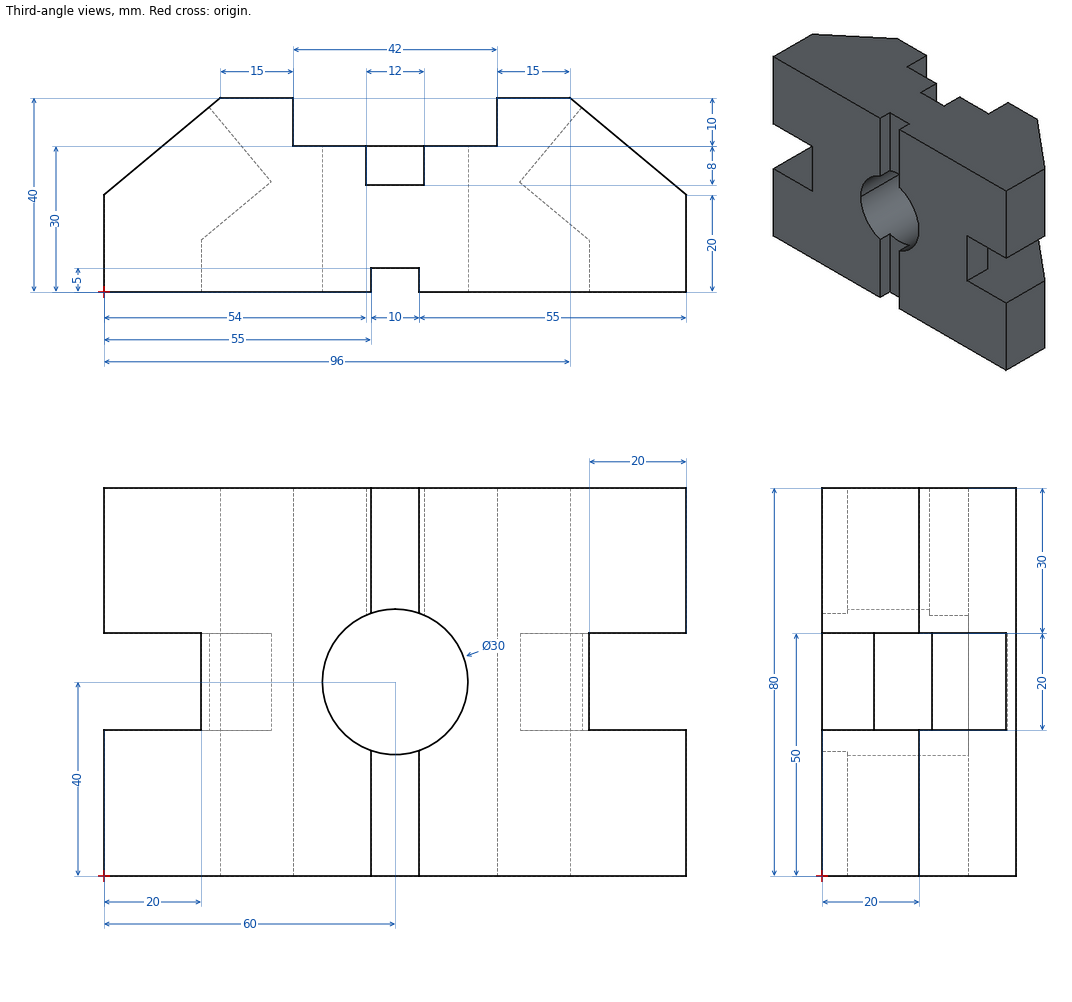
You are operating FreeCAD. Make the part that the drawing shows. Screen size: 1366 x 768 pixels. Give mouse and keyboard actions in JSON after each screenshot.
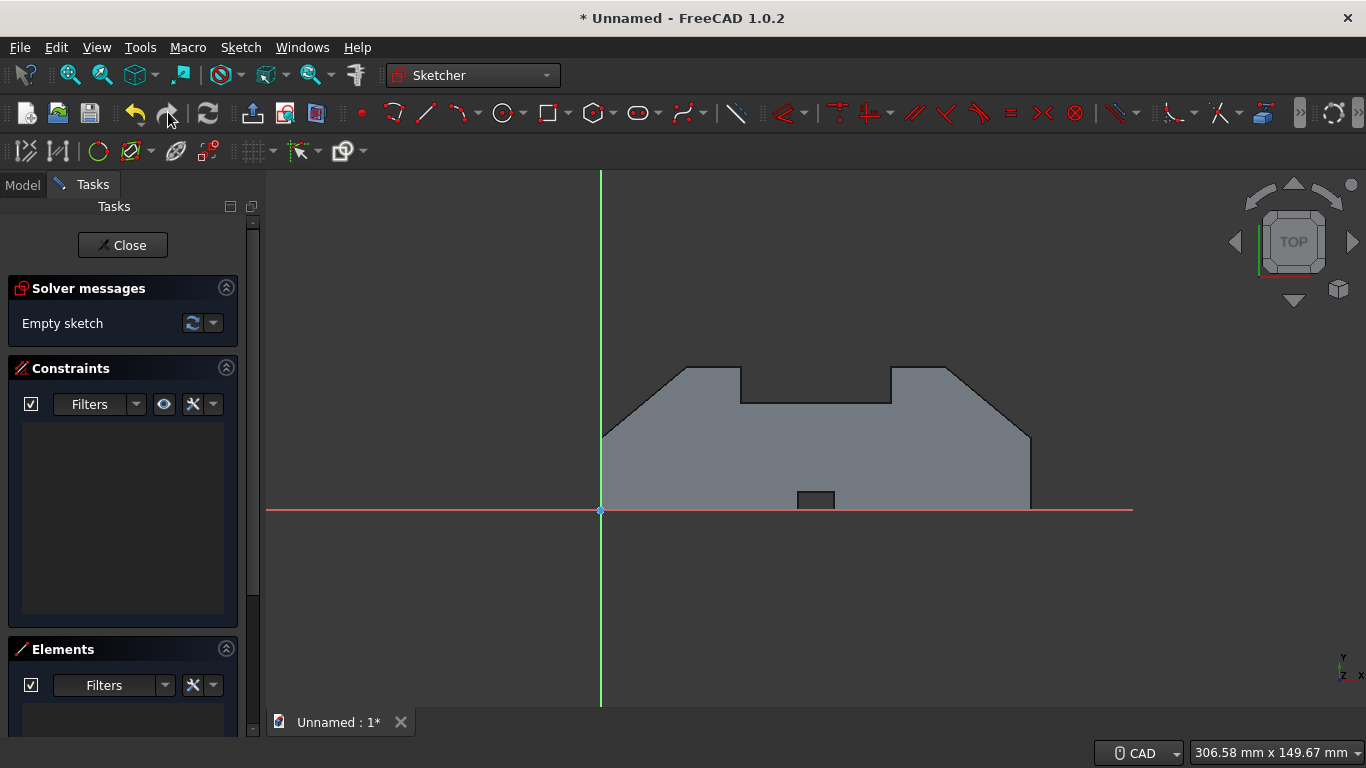
{"action": "scroll", "coordinate": [823, 415], "scroll_direction": "up", "scroll_amount": 12}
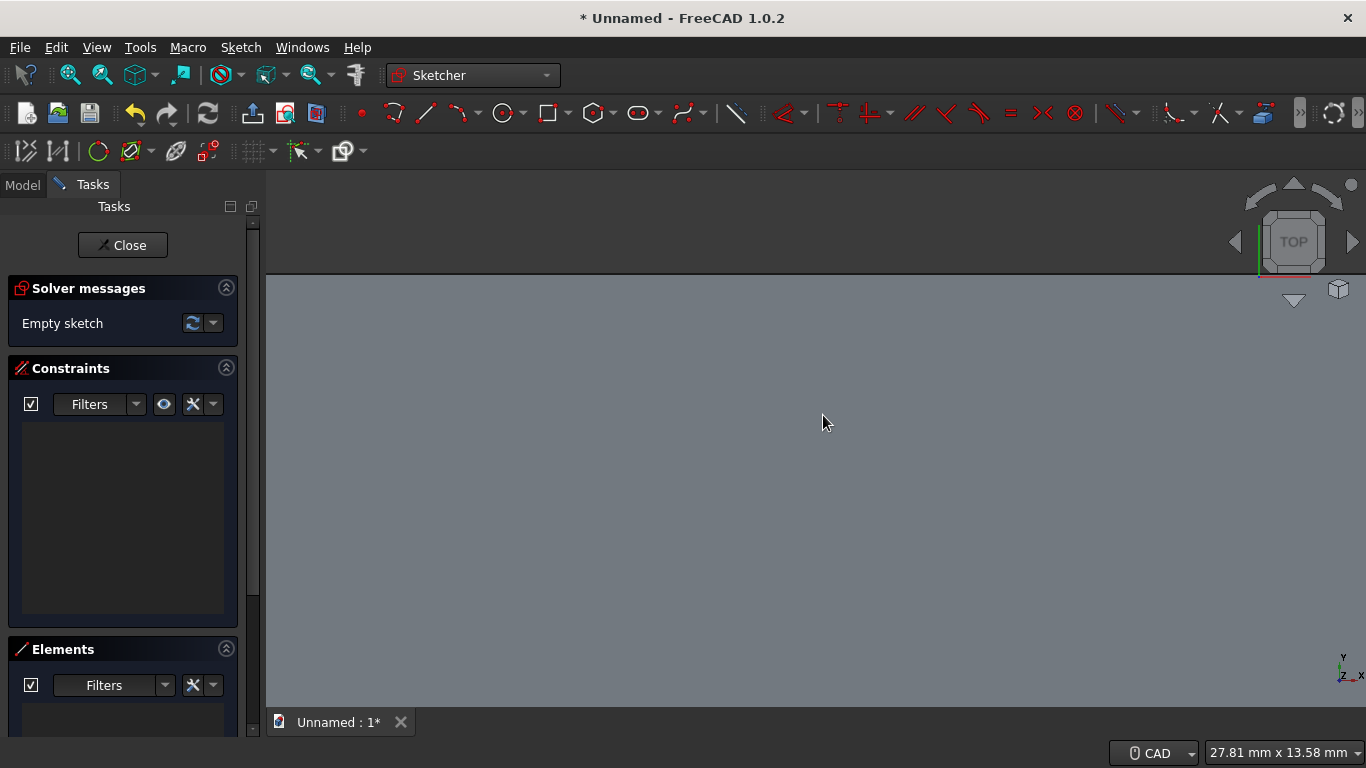
{"action": "key", "text": "g r"}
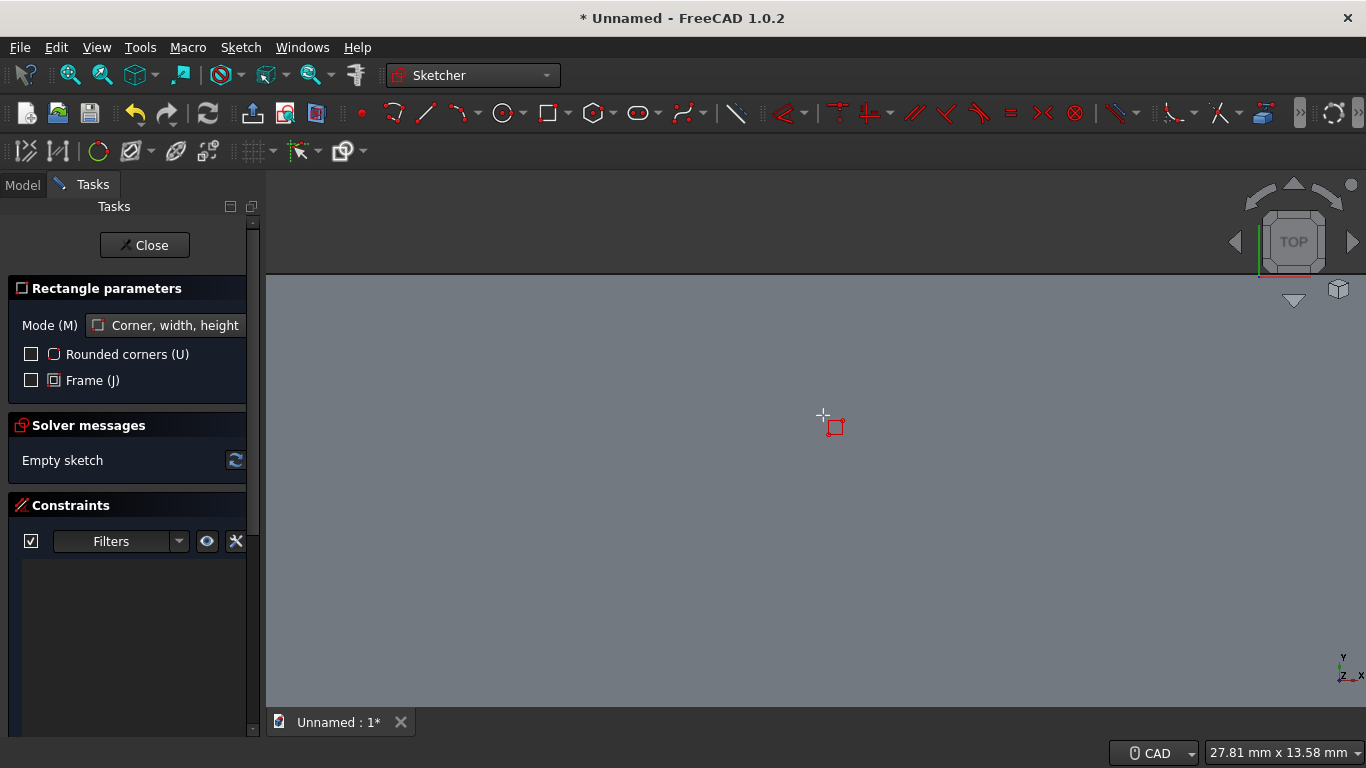
{"action": "left_click", "coordinate": [503, 274]}
{"action": "mouse_move", "coordinate": [978, 590]}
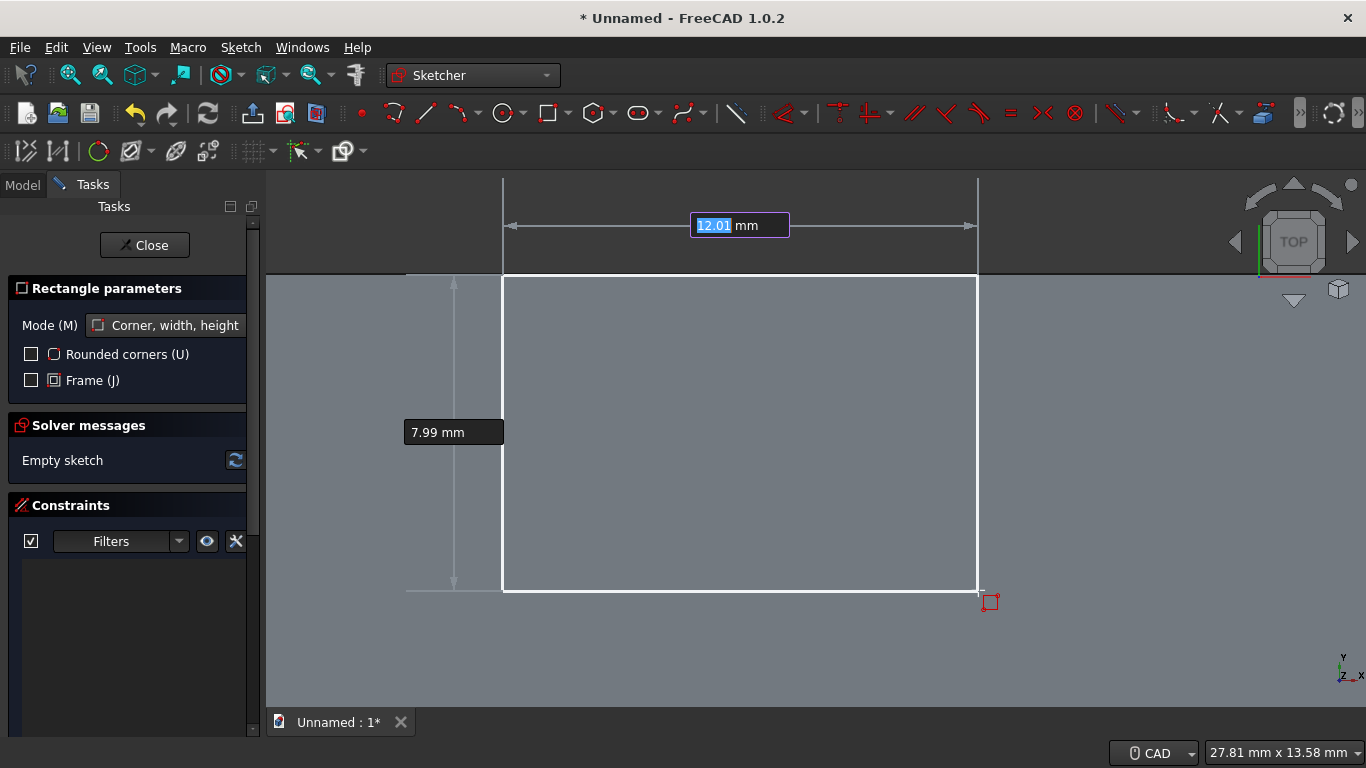
{"action": "type", "text": "12"}
{"action": "key", "text": "Tab"}
{"action": "type", "text": "8"}
{"action": "key", "text": "Return"}
{"action": "key", "text": "Escape"}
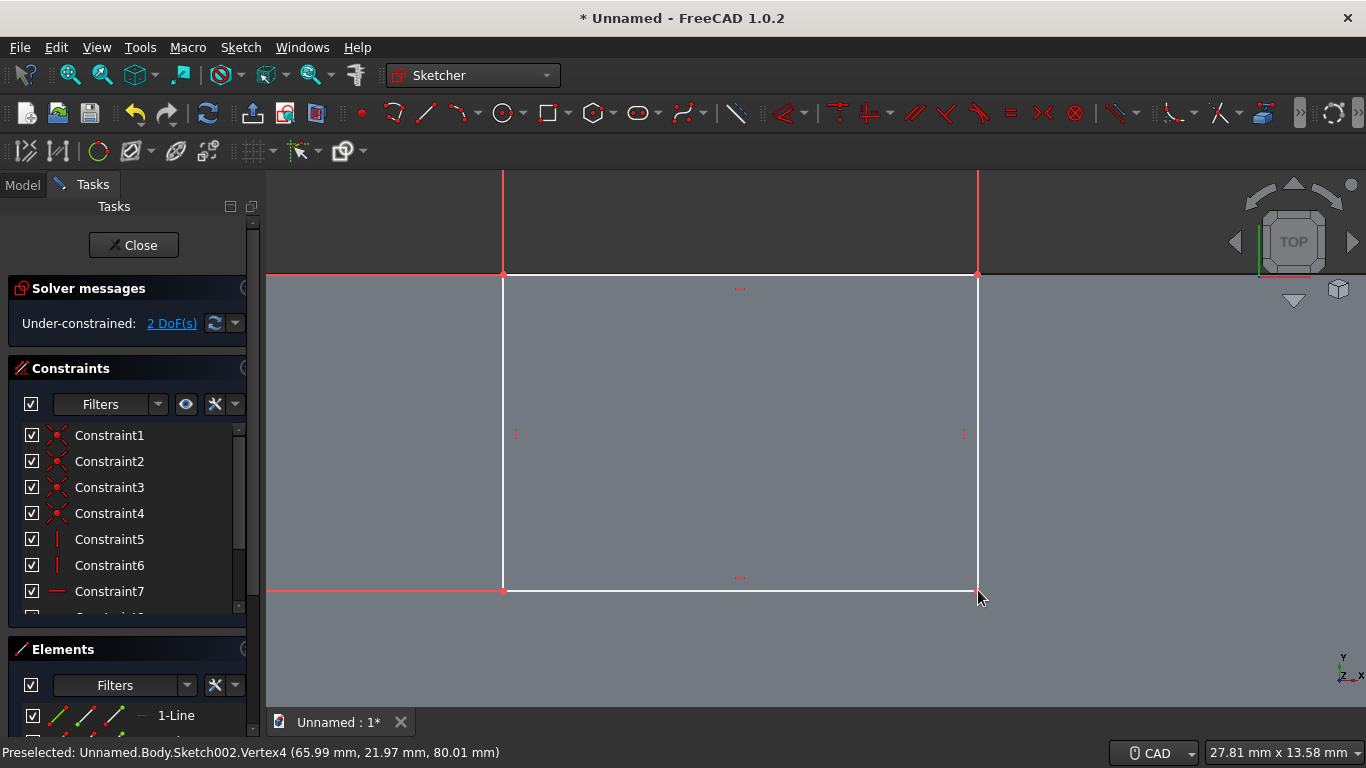
{"action": "key", "text": "d"}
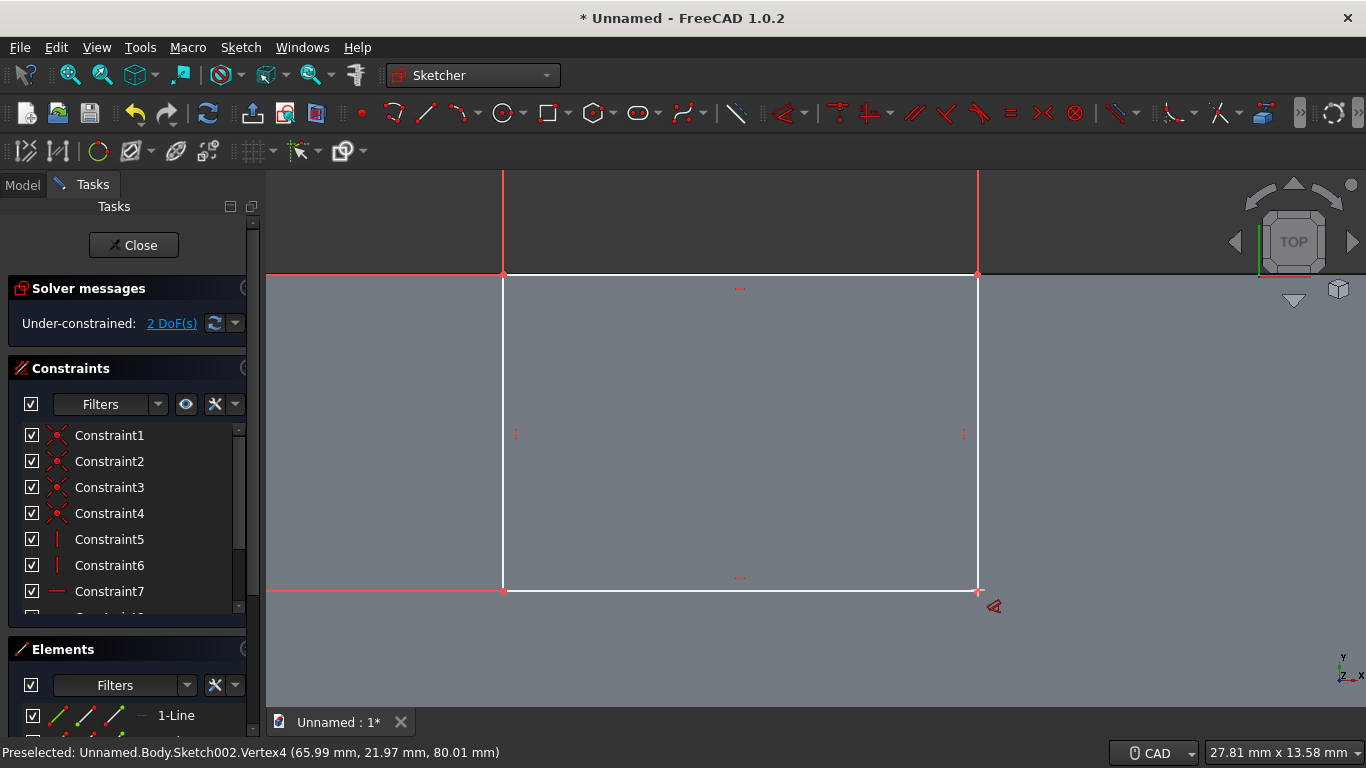
{"action": "left_click", "coordinate": [503, 275]}
{"action": "left_click", "coordinate": [399, 241]}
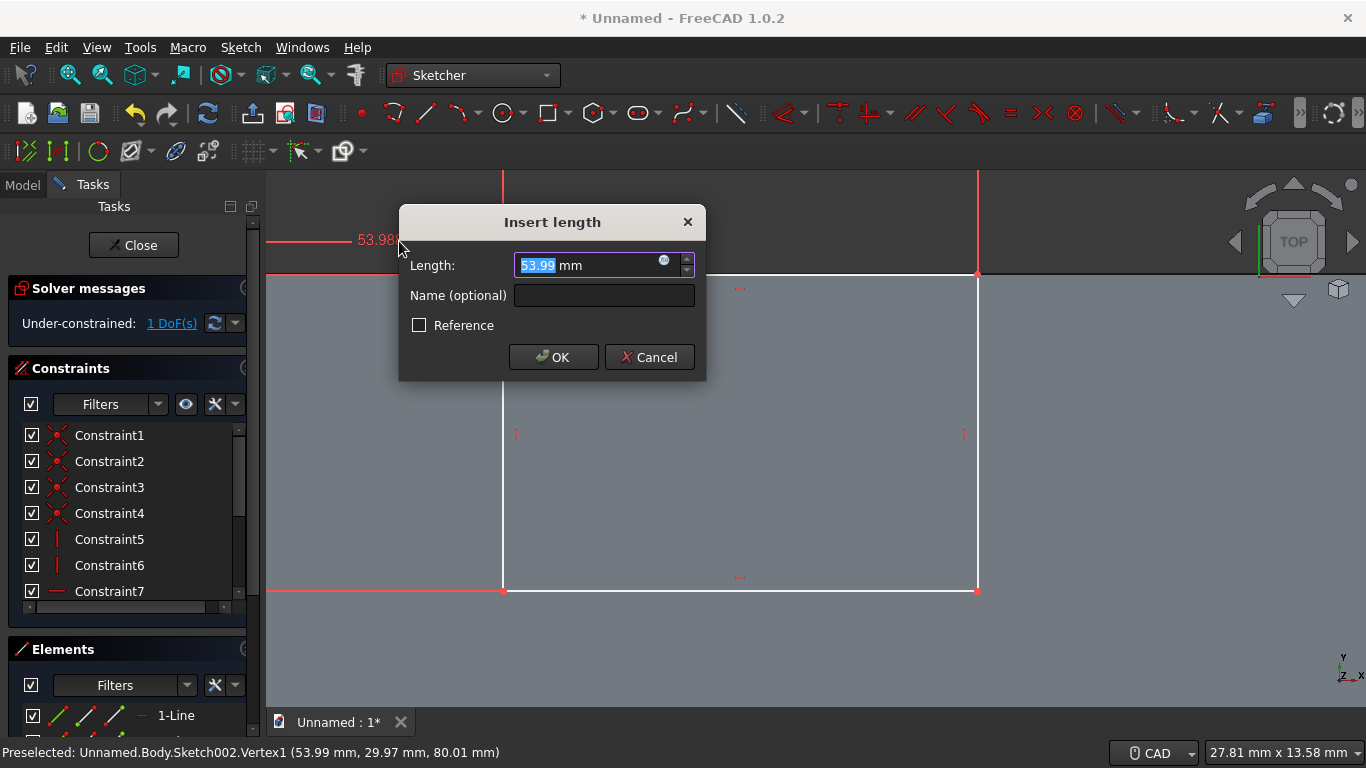
{"action": "type", "text": "54"}
{"action": "key", "text": "Return"}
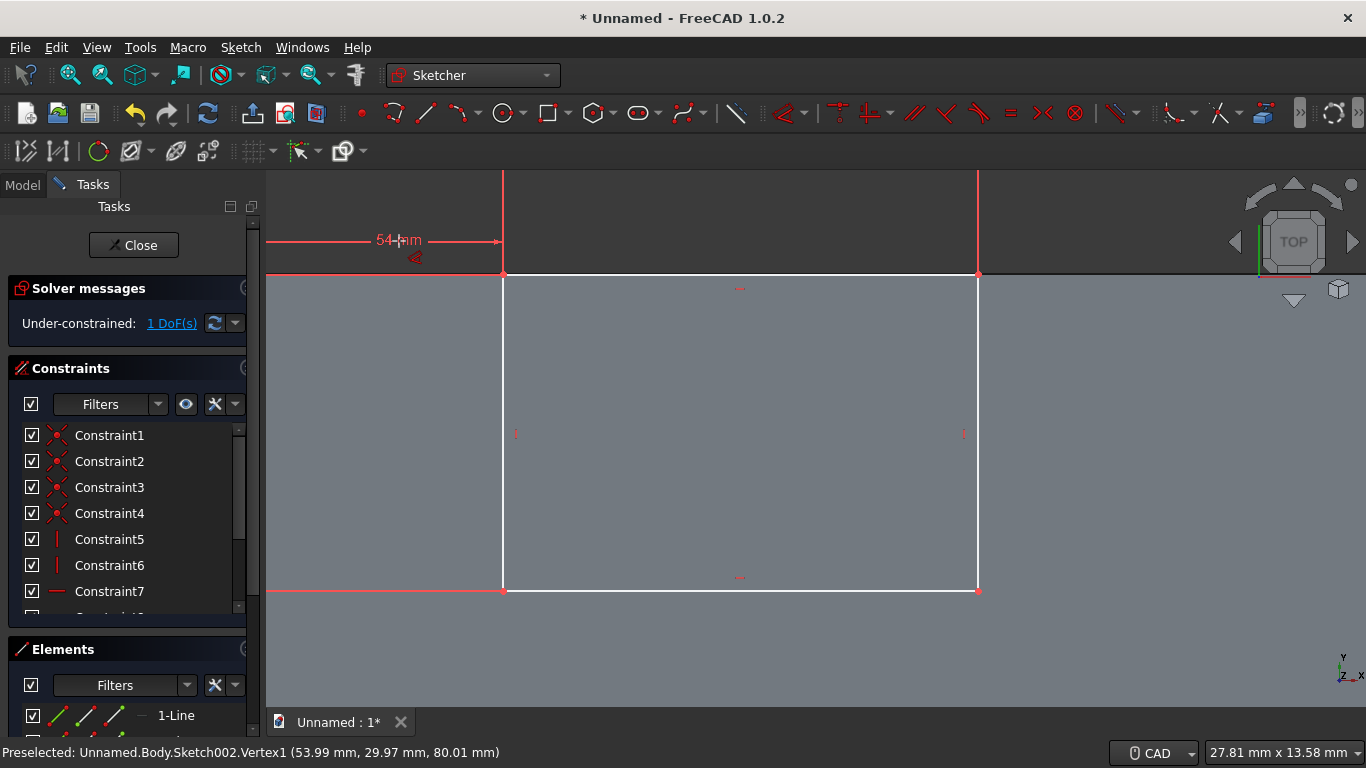
{"action": "left_click", "coordinate": [503, 275]}
{"action": "left_click", "coordinate": [537, 477]}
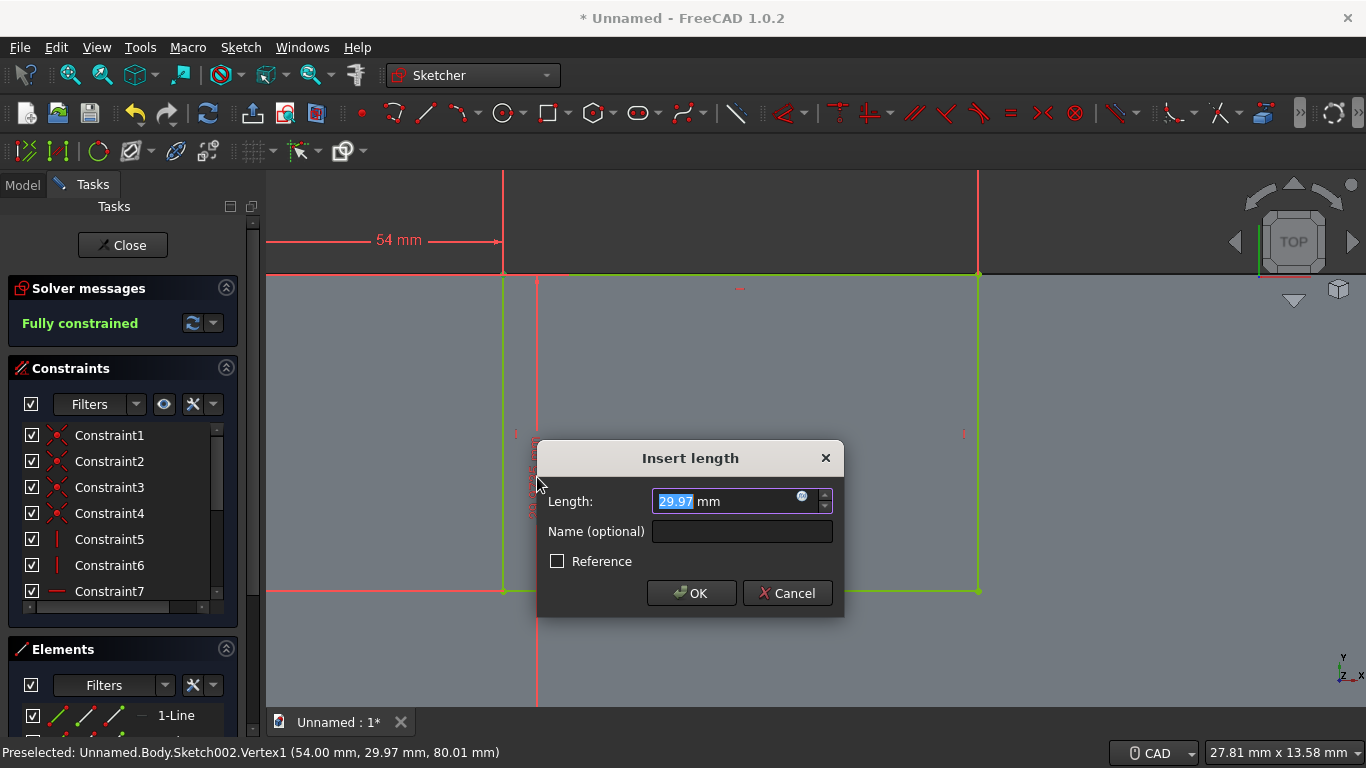
{"action": "type", "text": "30"}
{"action": "key", "text": "Return"}
{"action": "key", "text": "Escape"}